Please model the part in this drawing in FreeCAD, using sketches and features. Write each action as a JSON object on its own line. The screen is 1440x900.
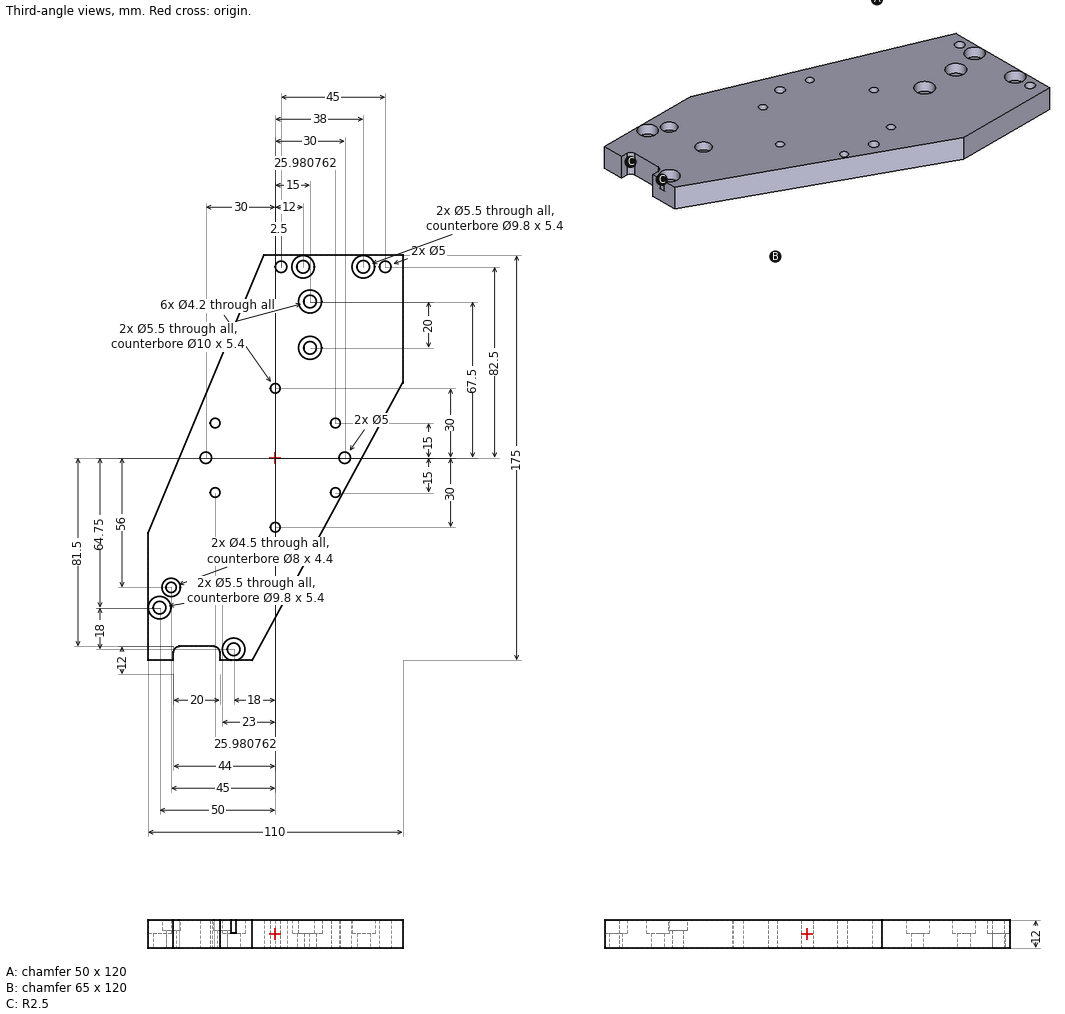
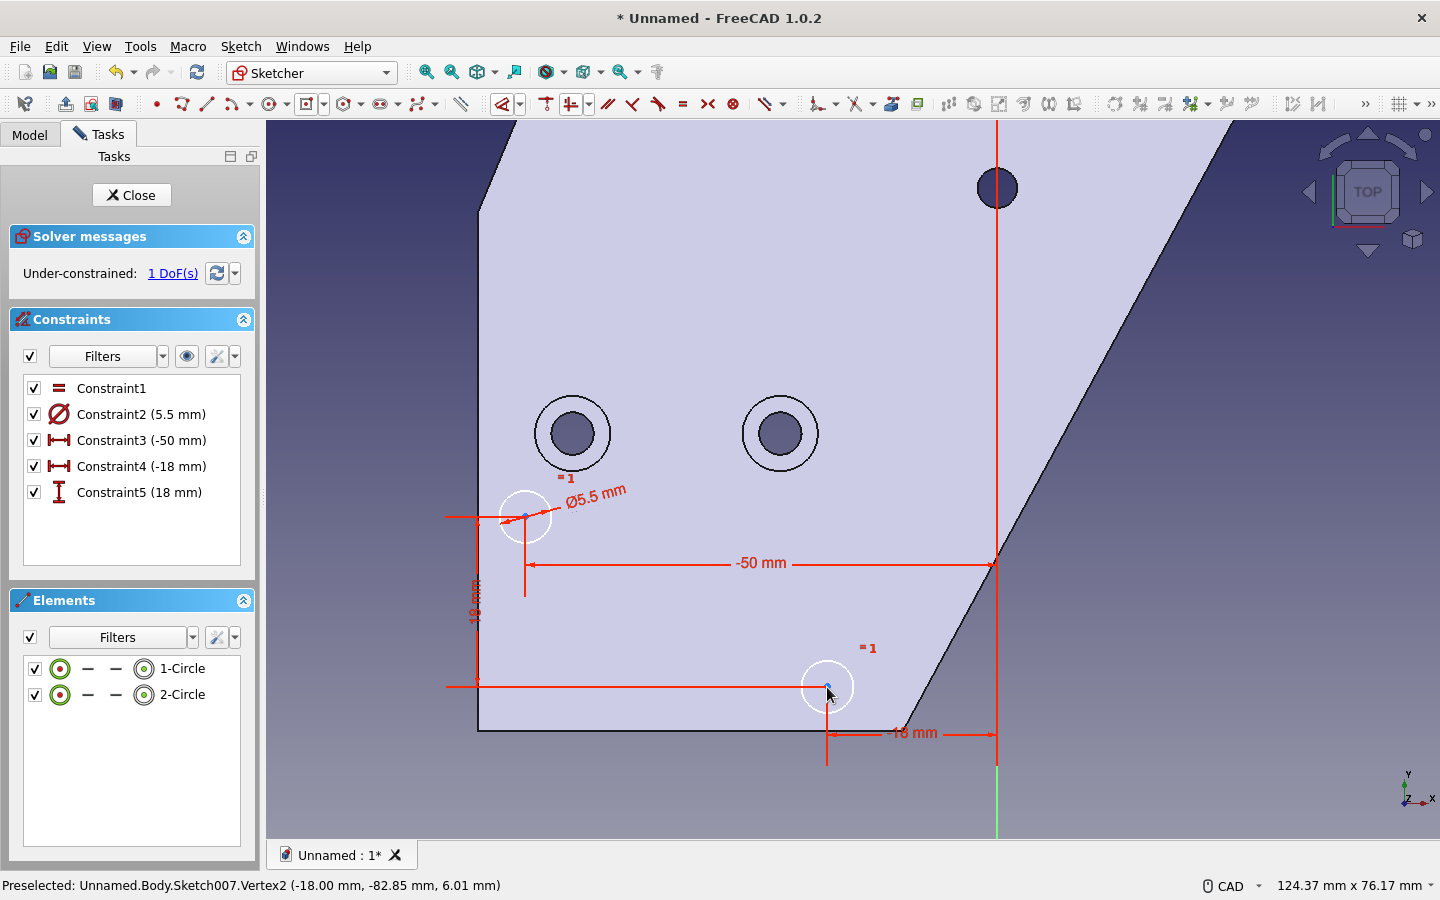
{"action": "left_click", "coordinate": [525, 517]}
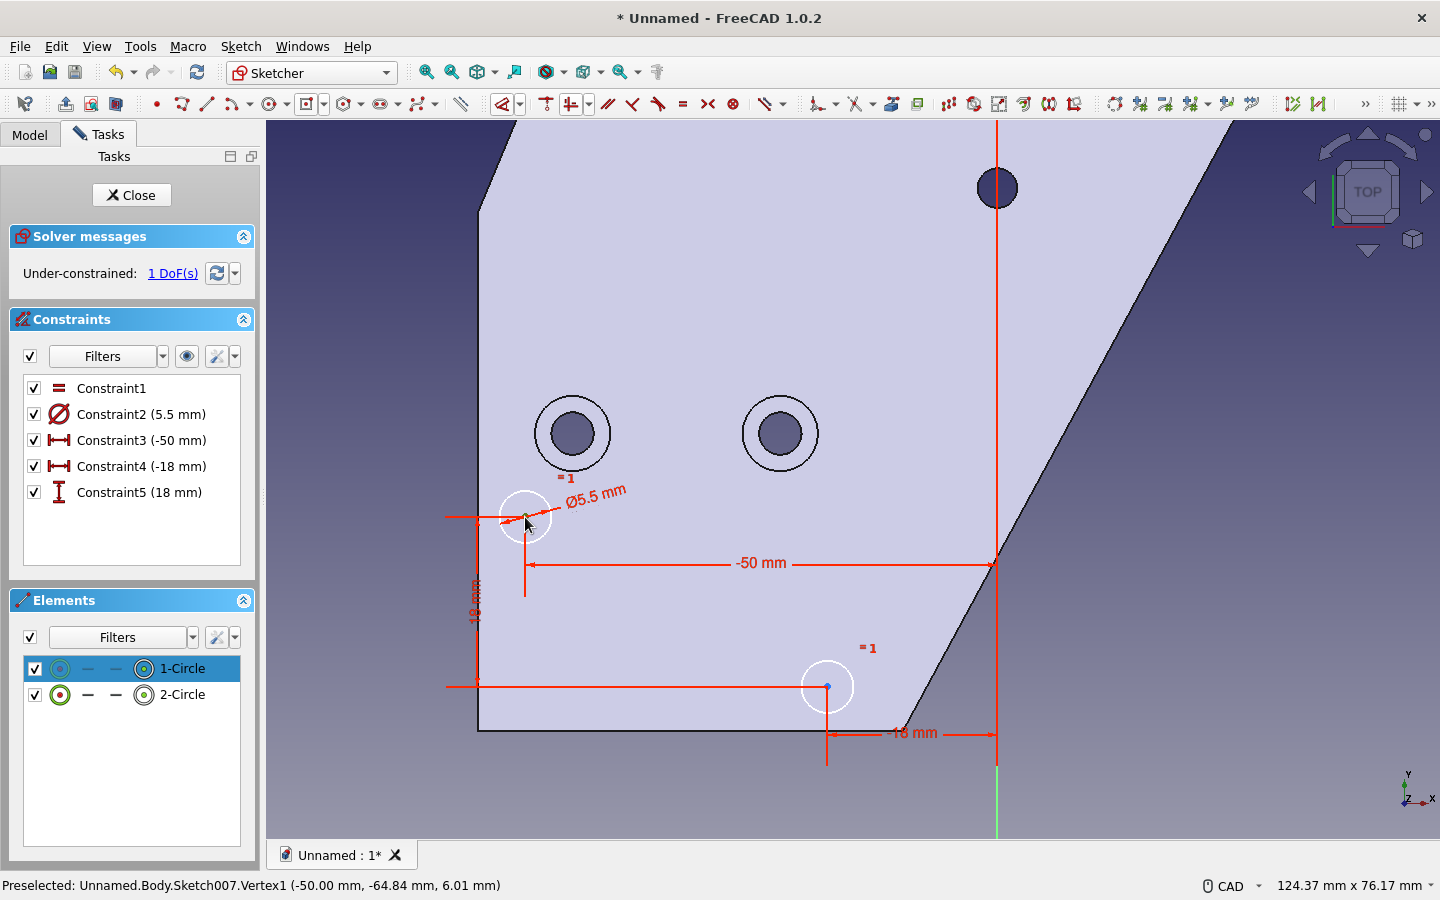
{"action": "key", "text": "i"}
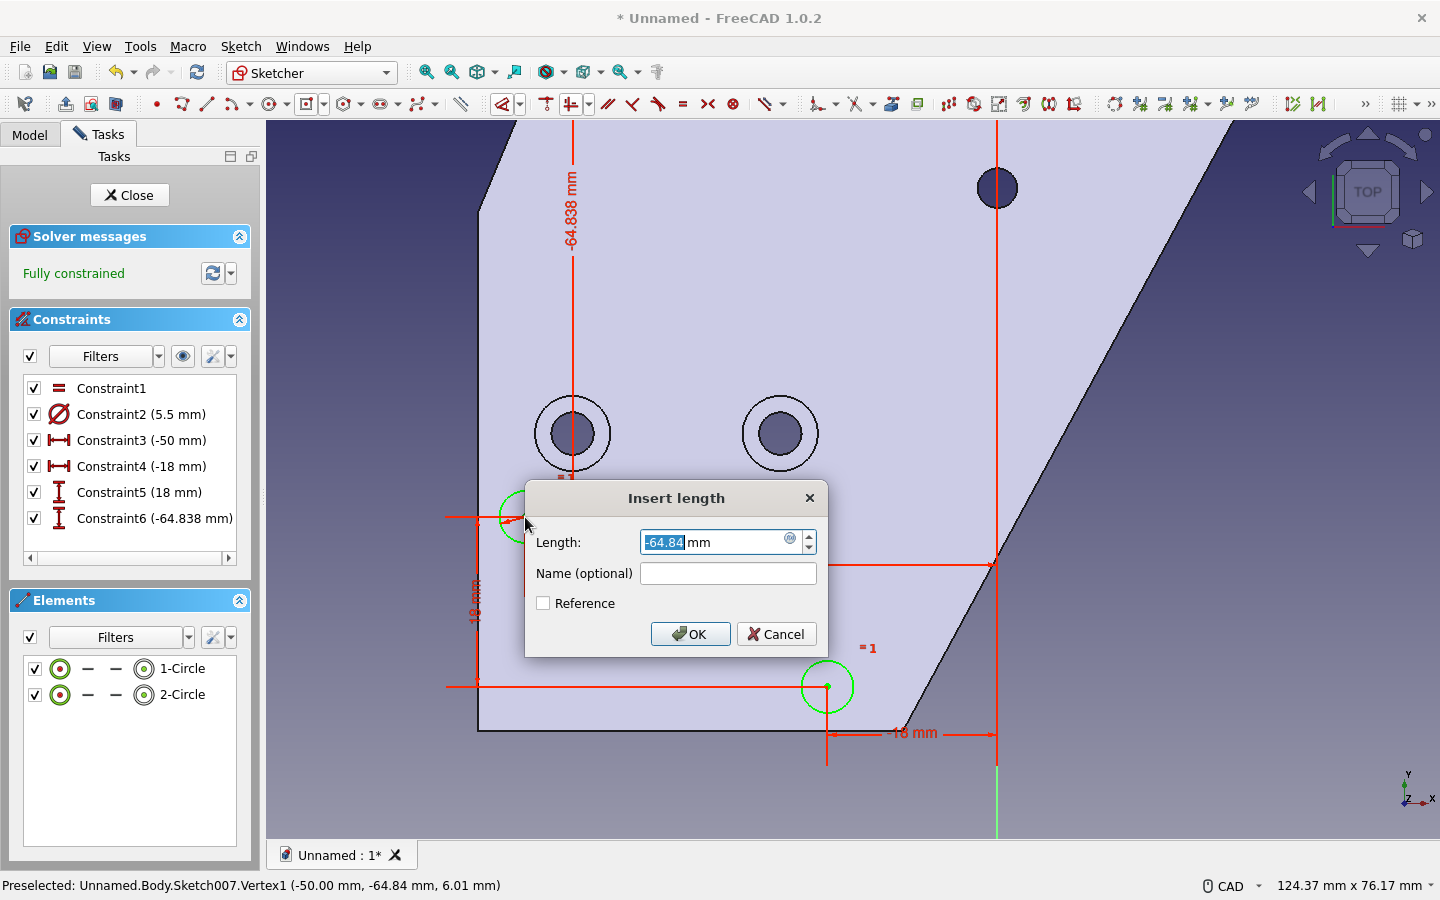
{"action": "type", "text": "-64.75"}
{"action": "key", "text": "Return"}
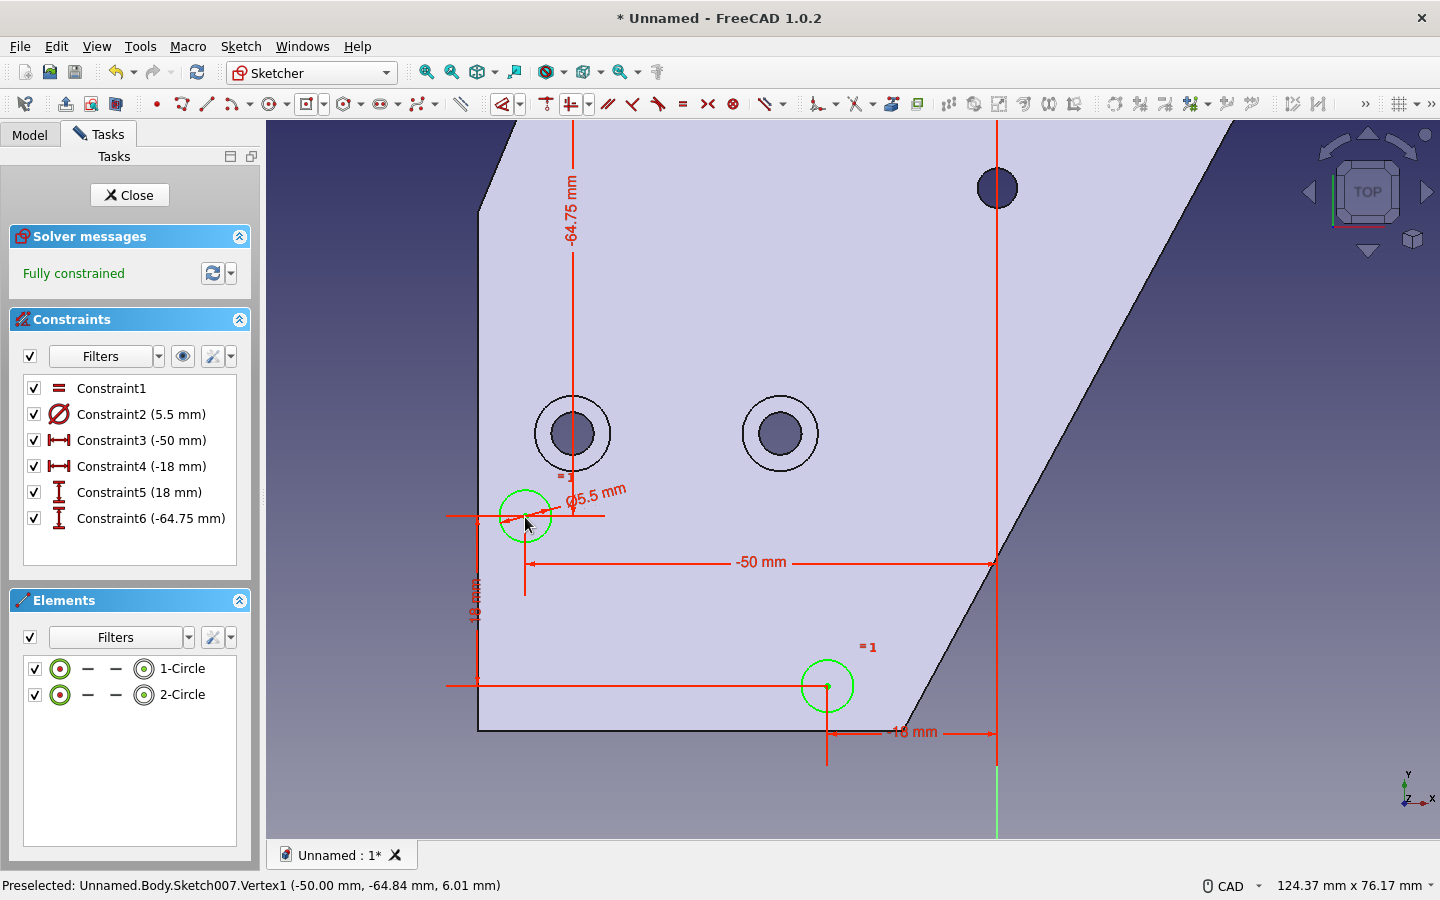
{"action": "left_click", "coordinate": [130, 195]}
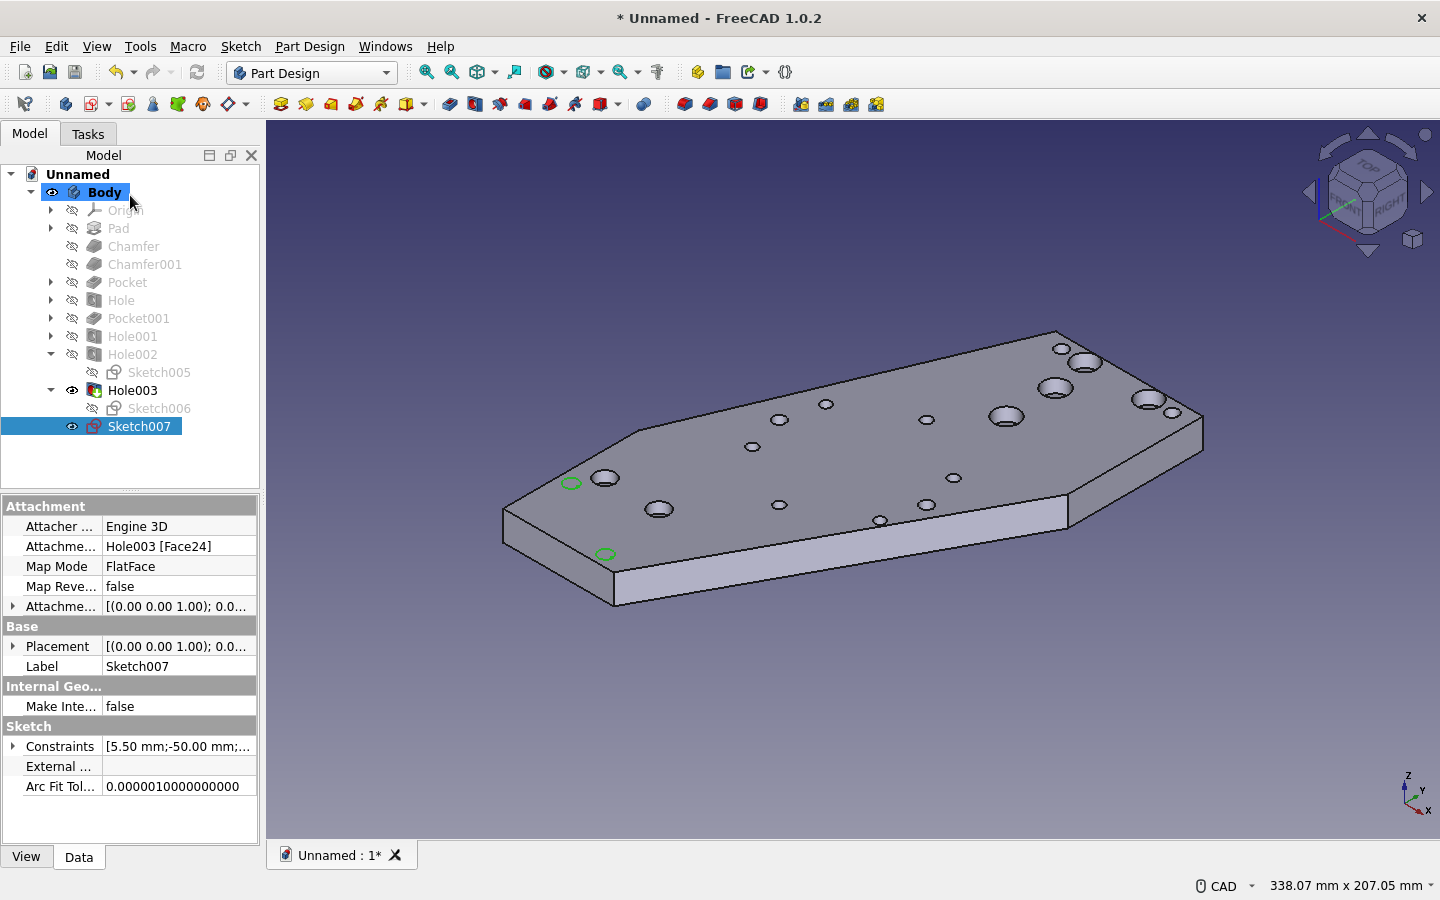
{"action": "left_click", "coordinate": [475, 104]}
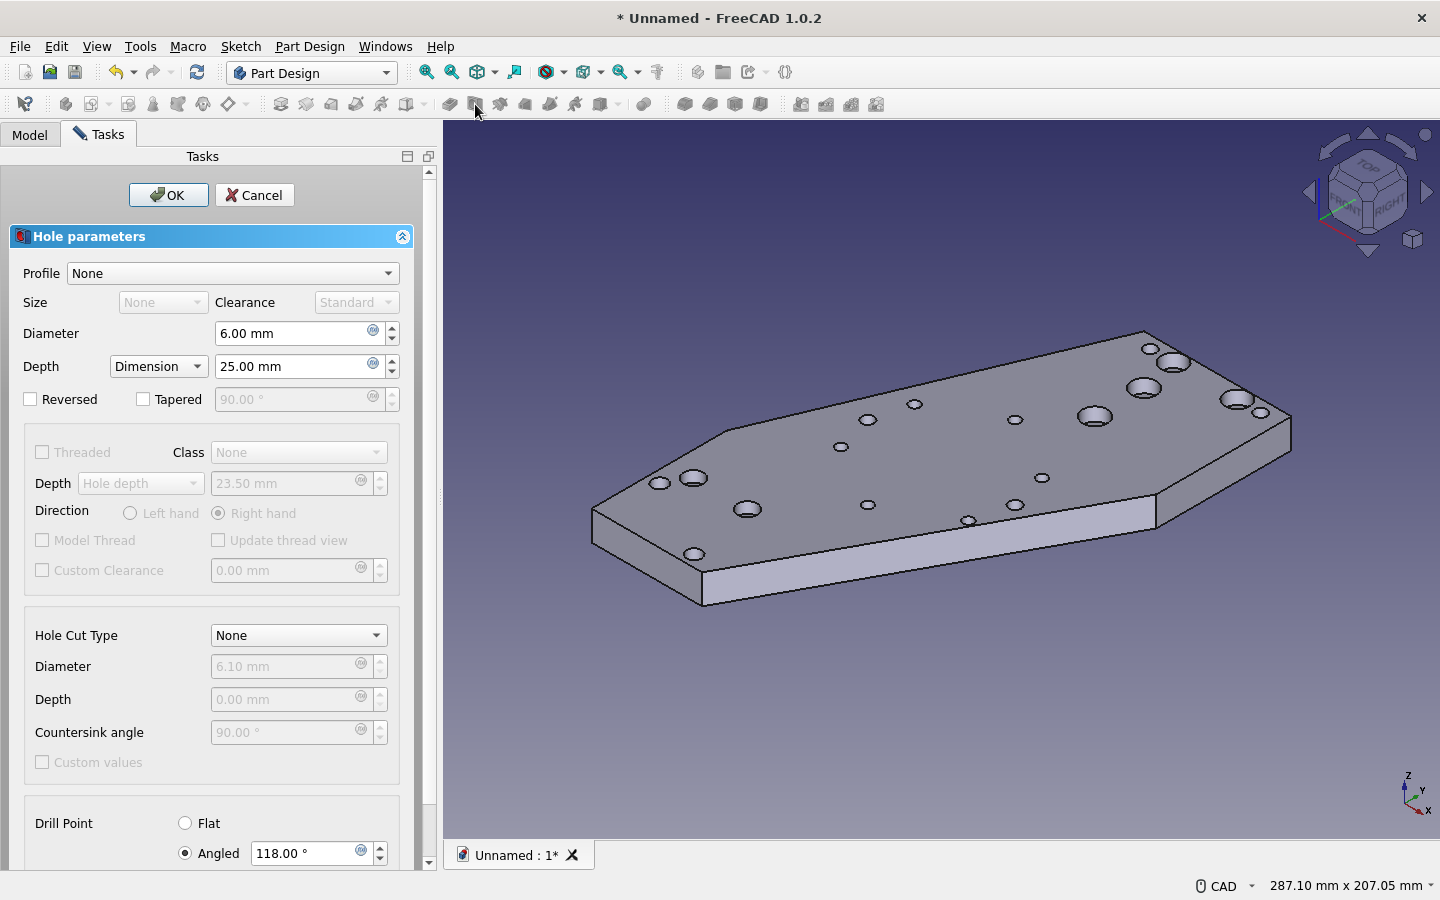
{"action": "triple_click", "coordinate": [300, 334]}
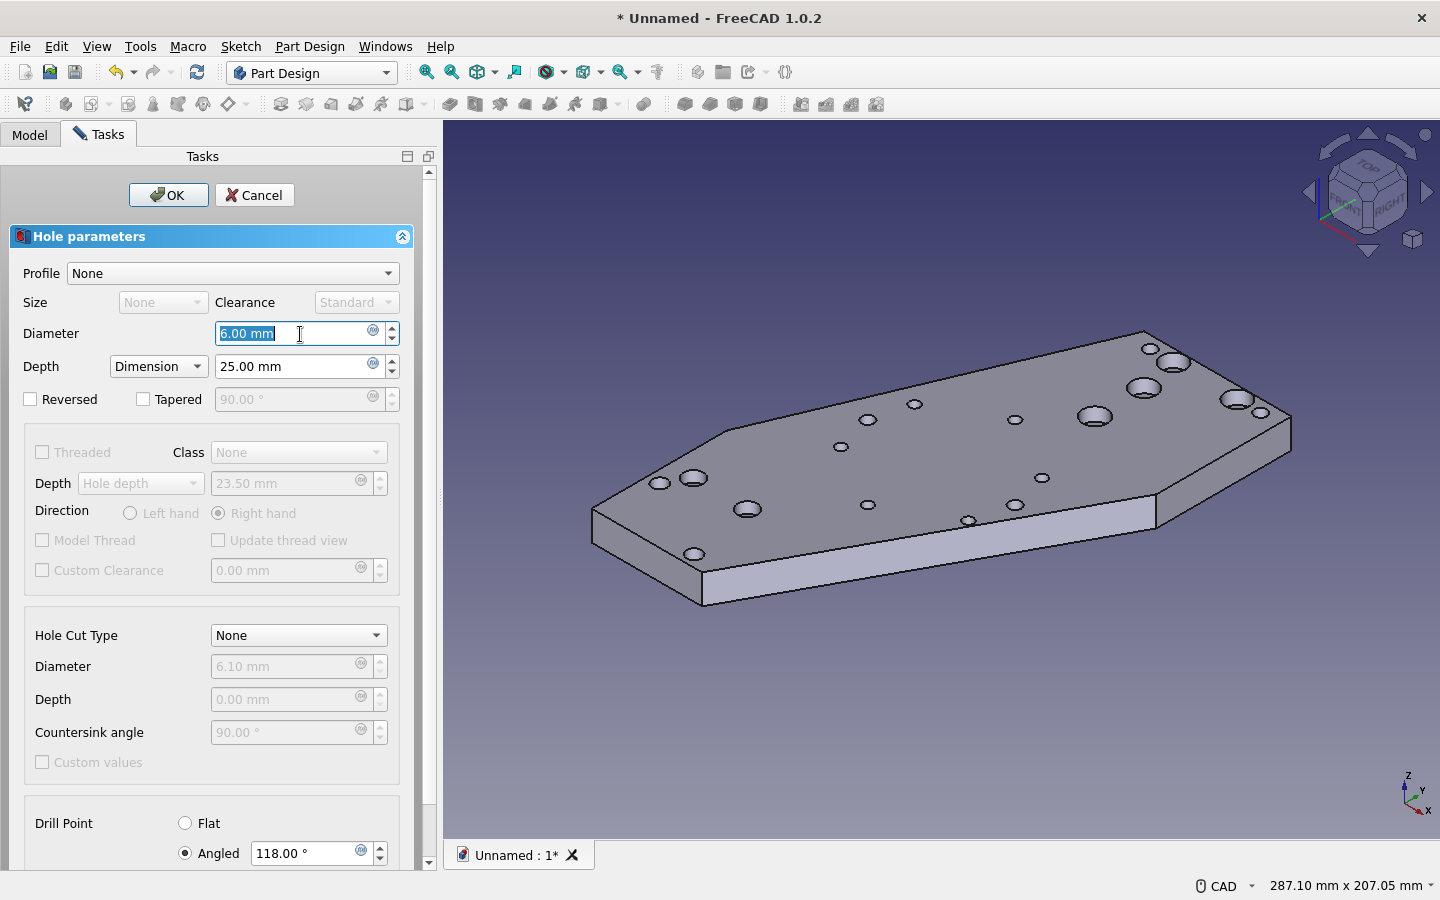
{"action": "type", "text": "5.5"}
{"action": "key", "text": "Tab"}